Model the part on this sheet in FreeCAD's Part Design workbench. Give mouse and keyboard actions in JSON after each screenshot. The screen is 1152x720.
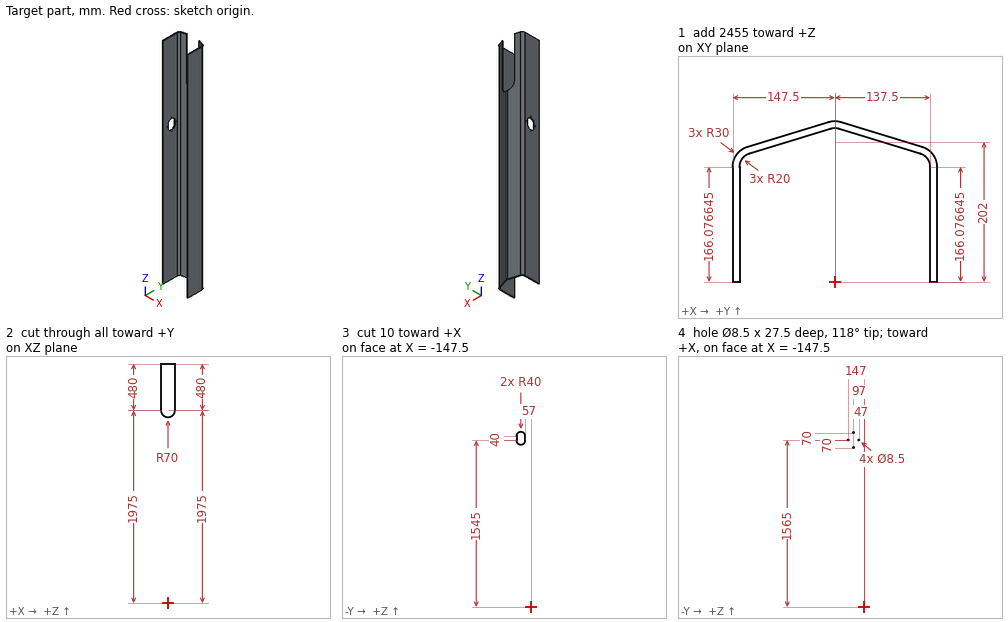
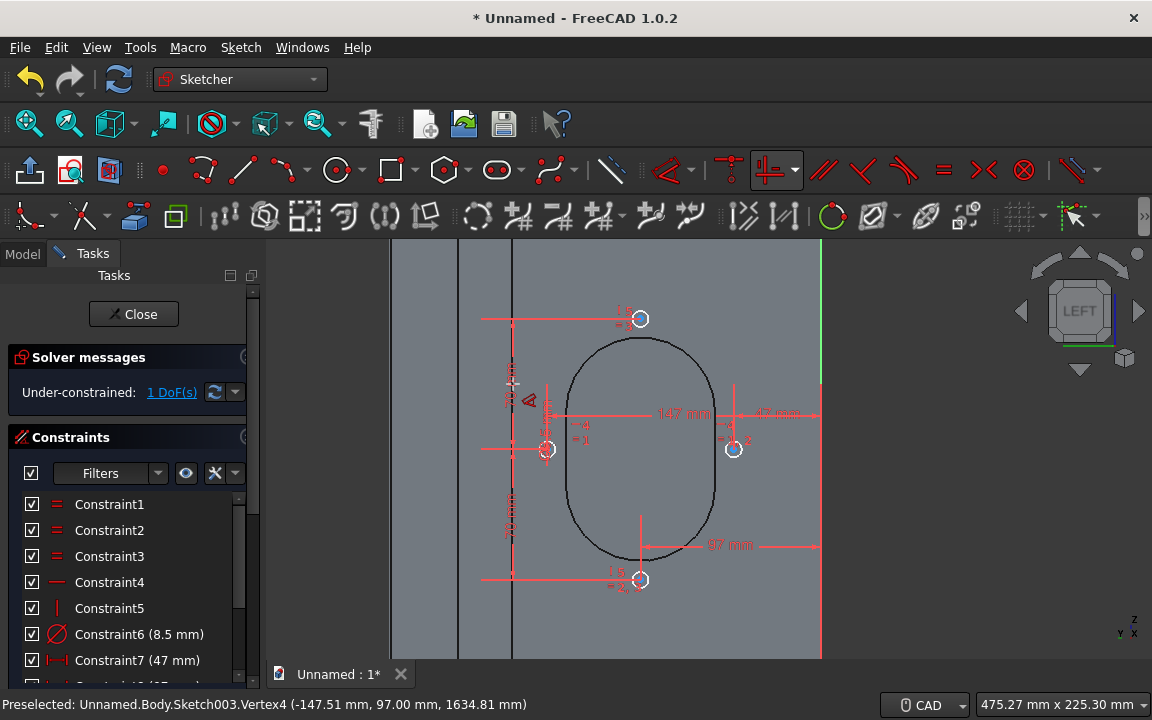
{"action": "left_click", "coordinate": [547, 449]}
{"action": "left_click", "coordinate": [855, 540]}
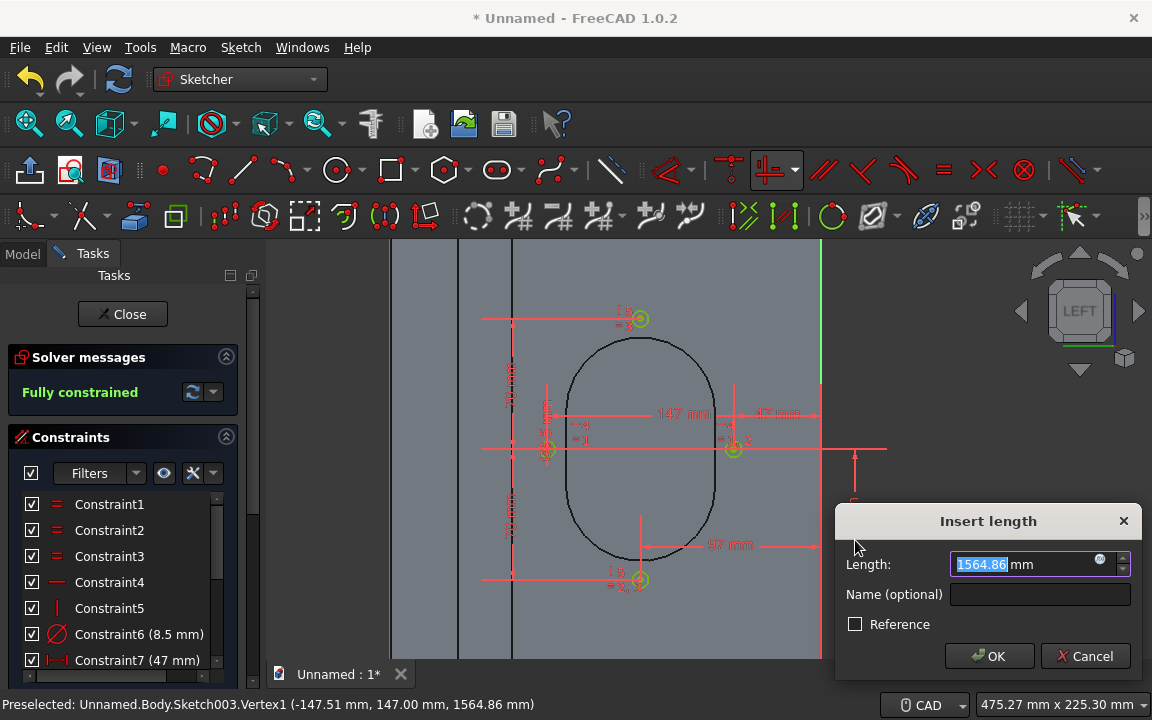
{"action": "type", "text": "1565"}
{"action": "key", "text": "Return"}
{"action": "key", "text": "Escape"}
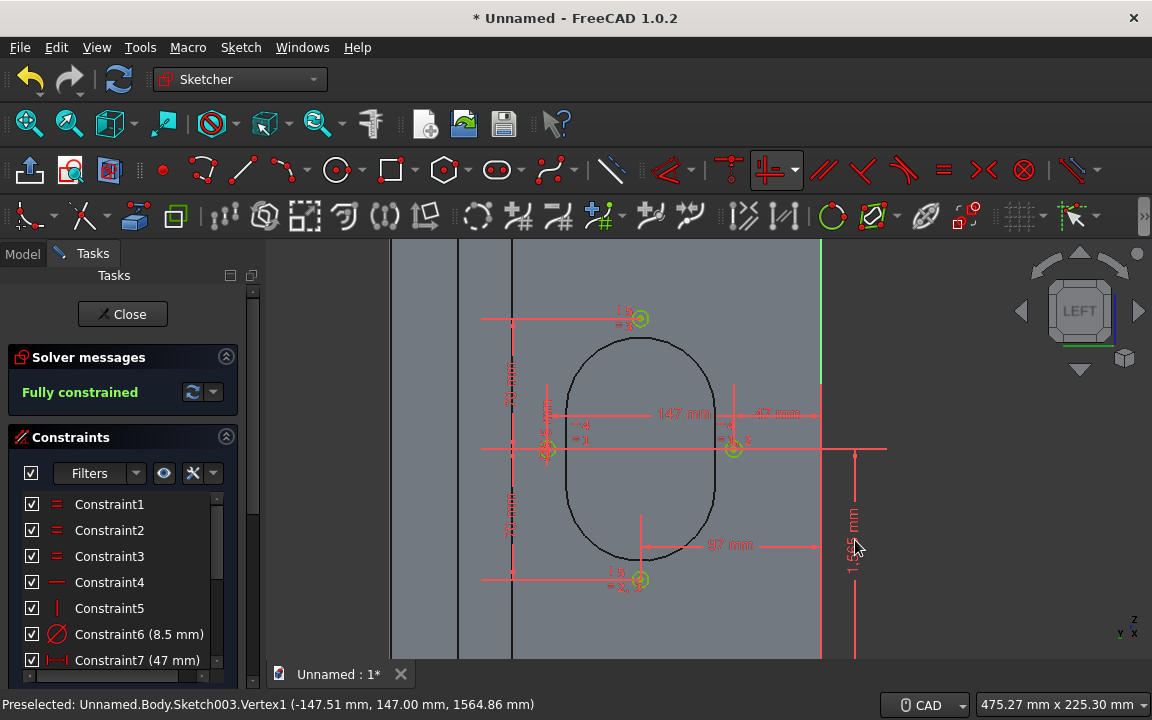
{"action": "left_click", "coordinate": [123, 314]}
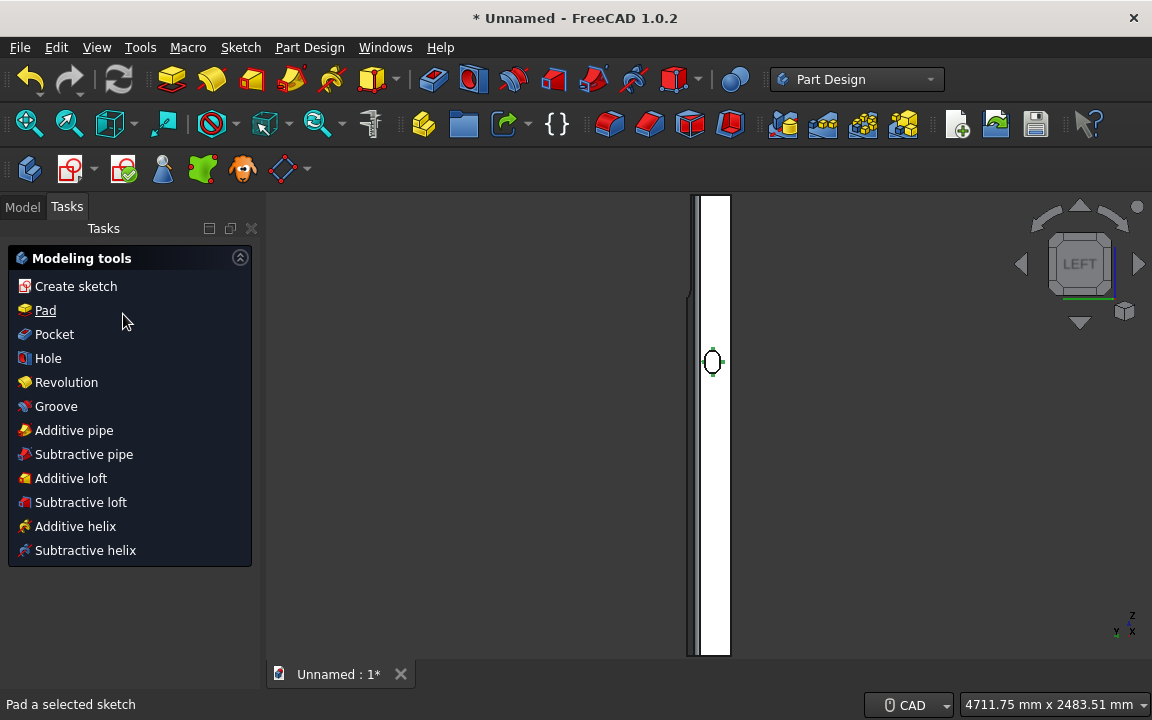
{"action": "left_click", "coordinate": [474, 80]}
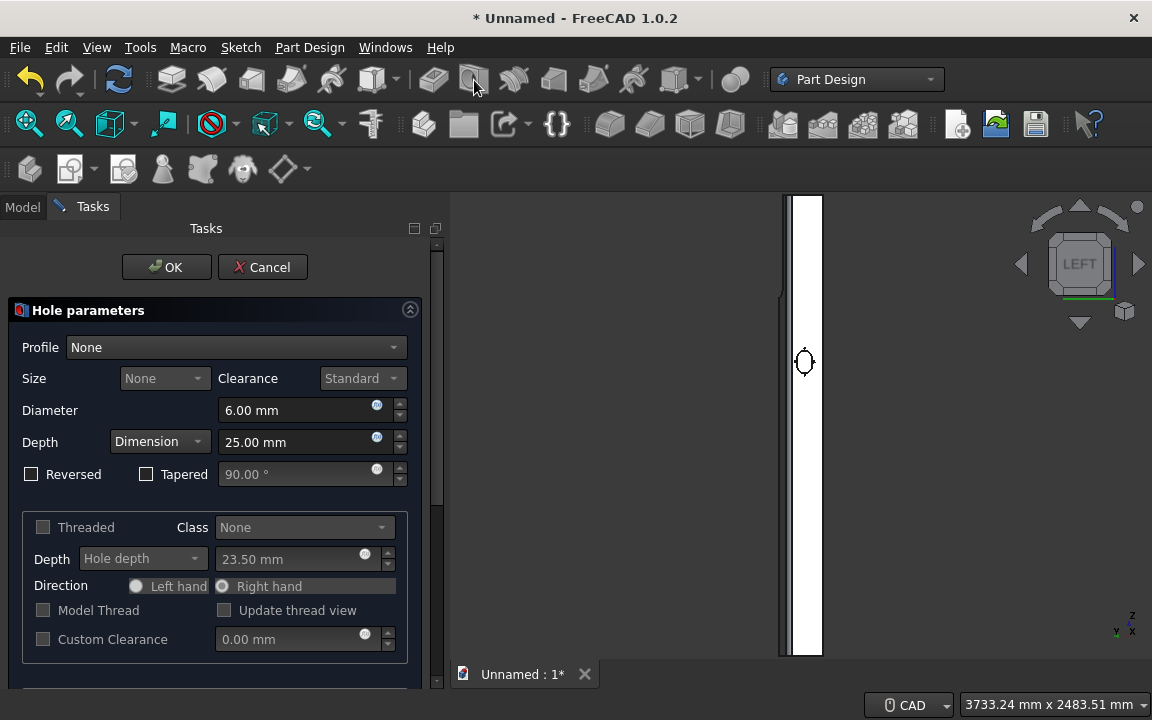
{"action": "triple_click", "coordinate": [305, 410]}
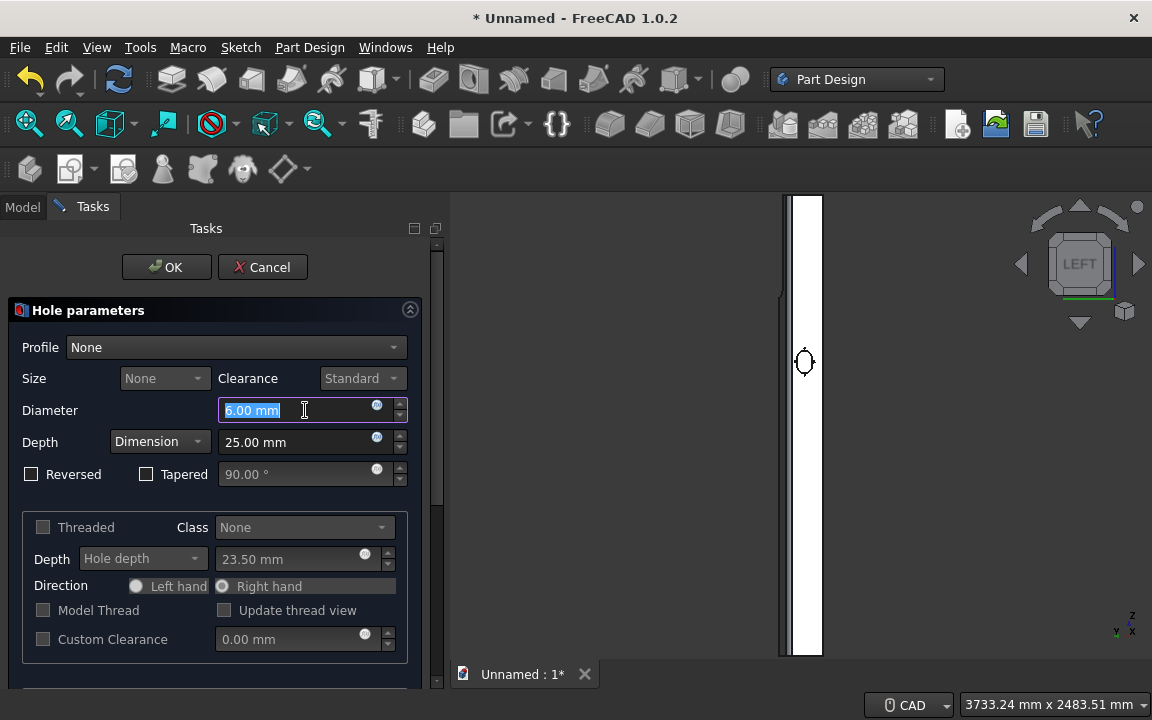
{"action": "type", "text": "8.5"}
{"action": "key", "text": "Tab"}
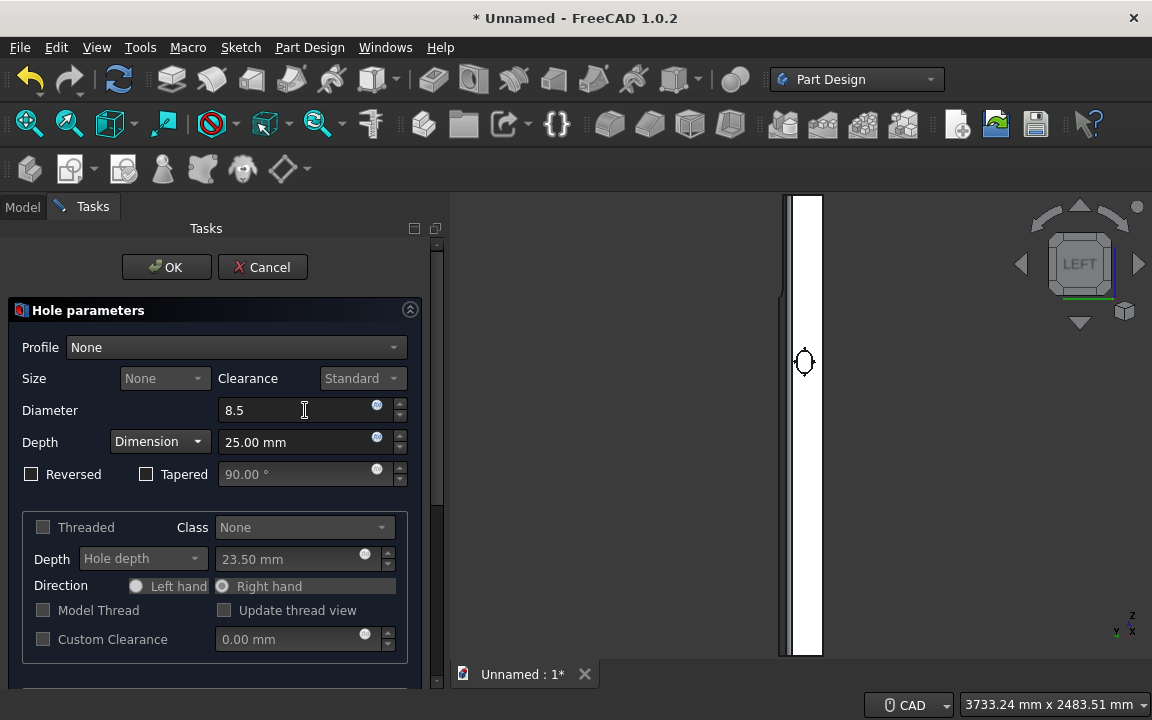
{"action": "triple_click", "coordinate": [305, 442]}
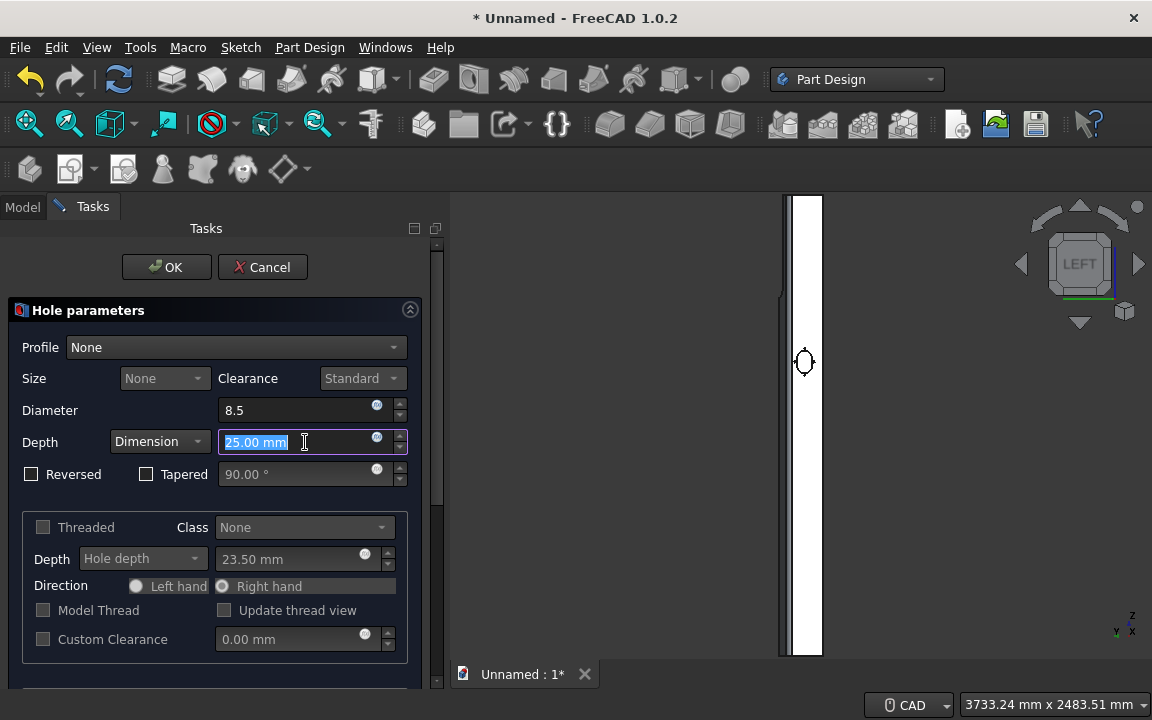
{"action": "type", "text": "27.5"}
{"action": "key", "text": "Tab"}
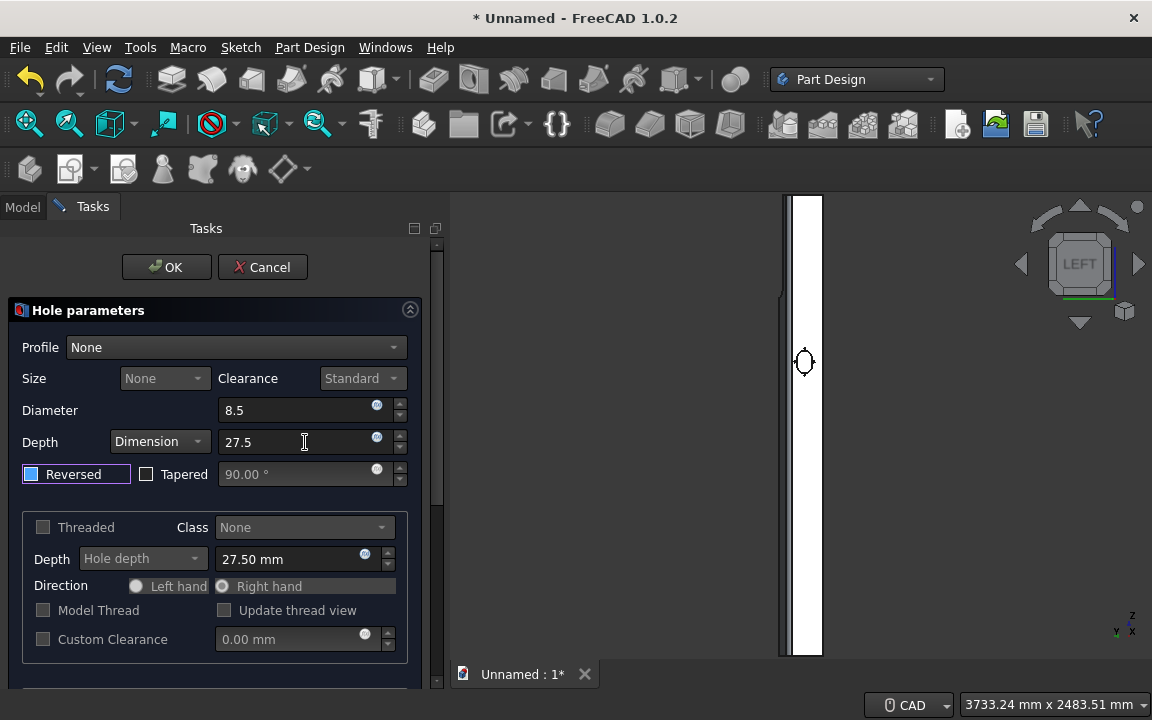
{"action": "left_click", "coordinate": [167, 267]}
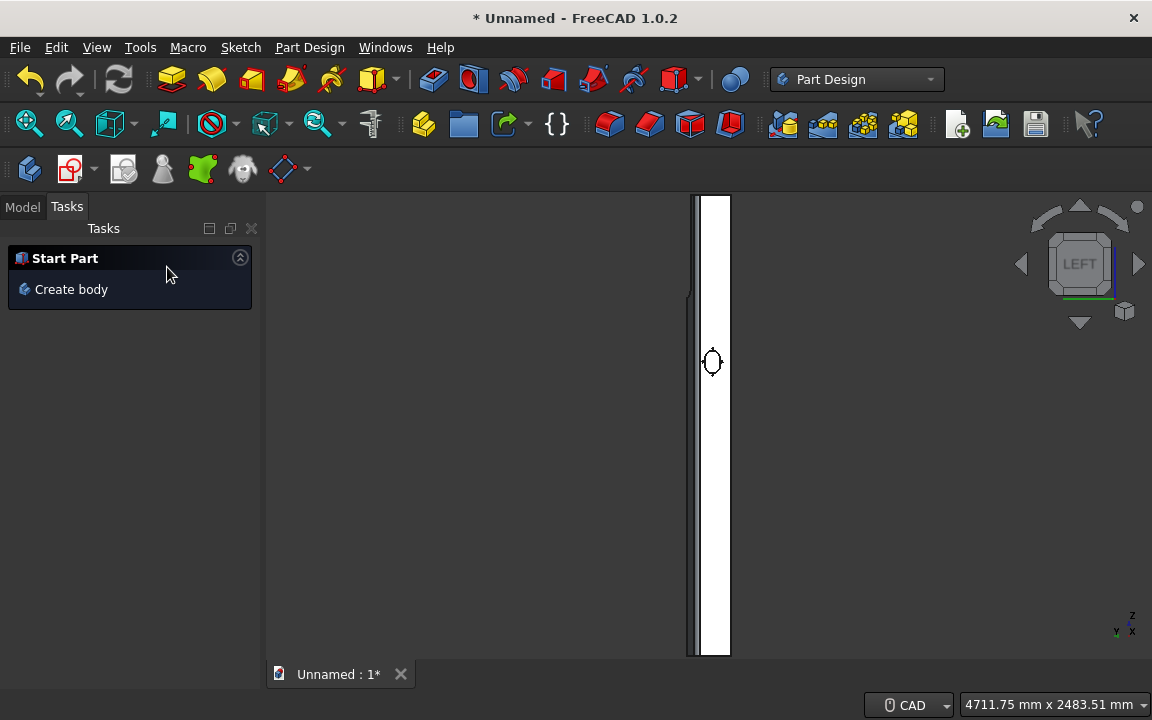
{"action": "key", "text": "0"}